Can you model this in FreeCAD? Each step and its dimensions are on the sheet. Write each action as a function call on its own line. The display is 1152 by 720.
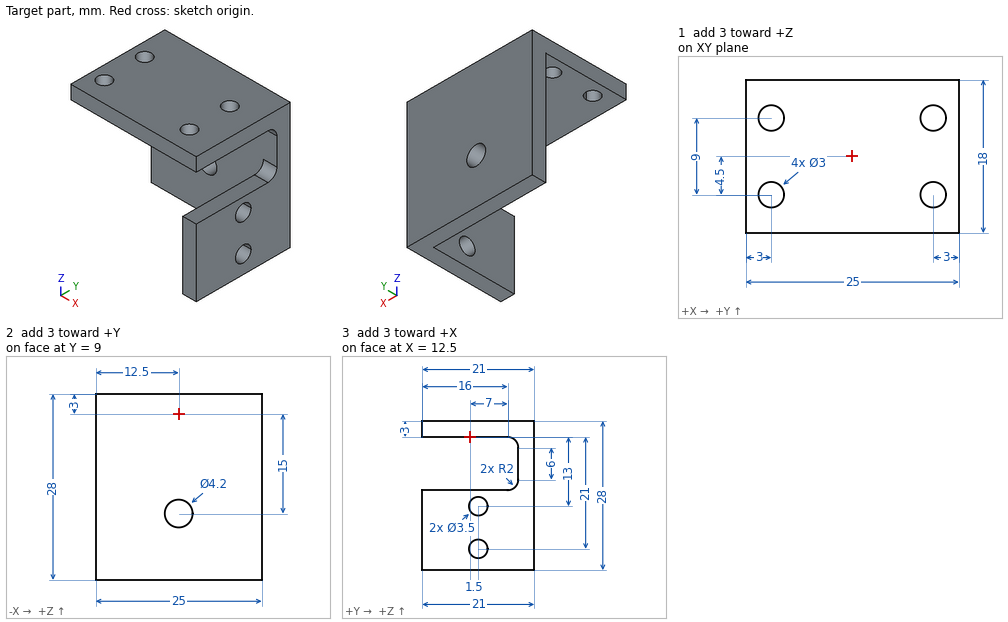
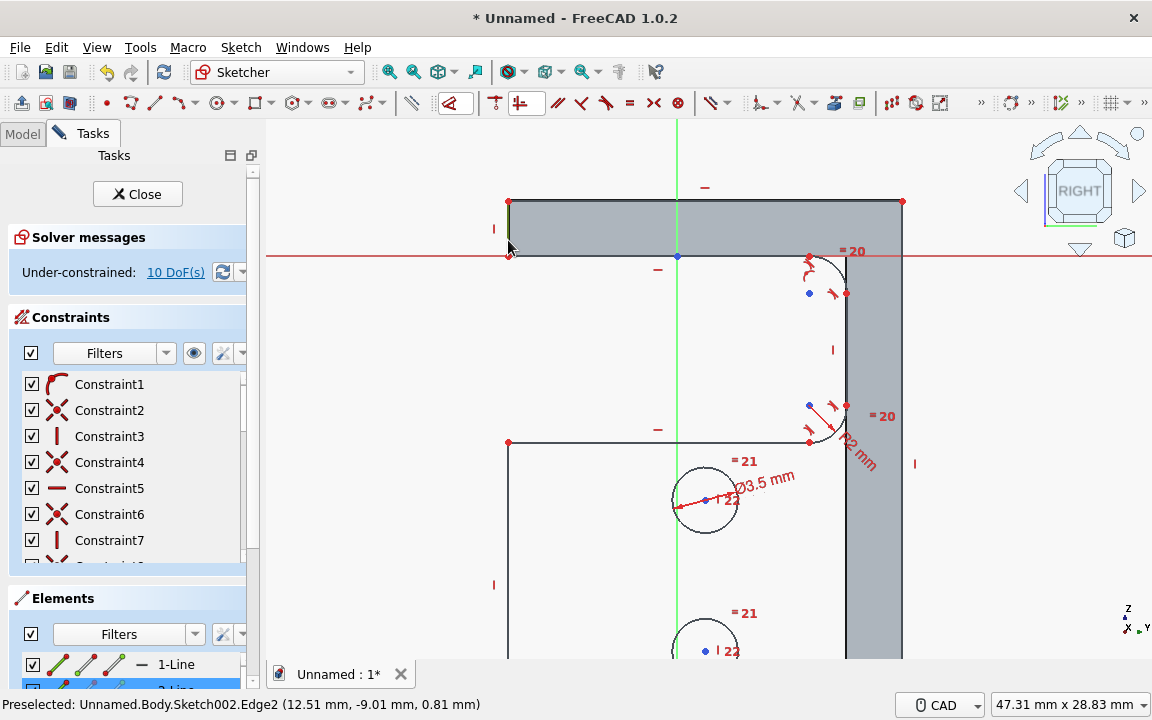
key(i)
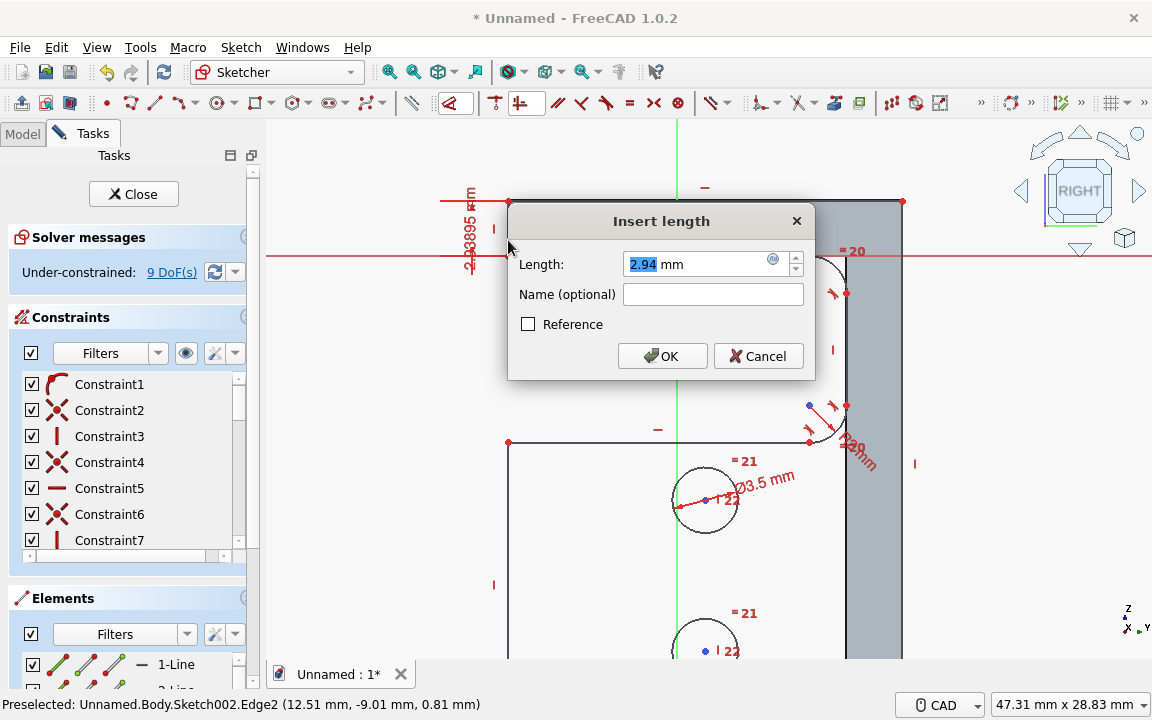
text(3)
key(Return)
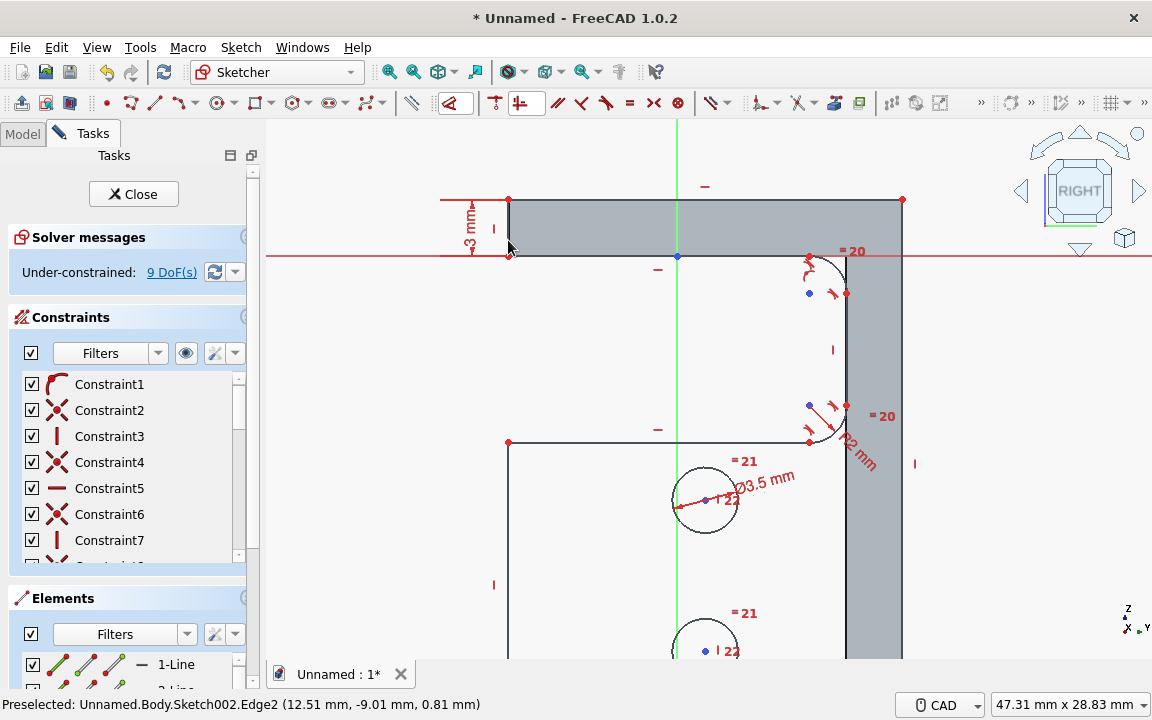
click(847, 372)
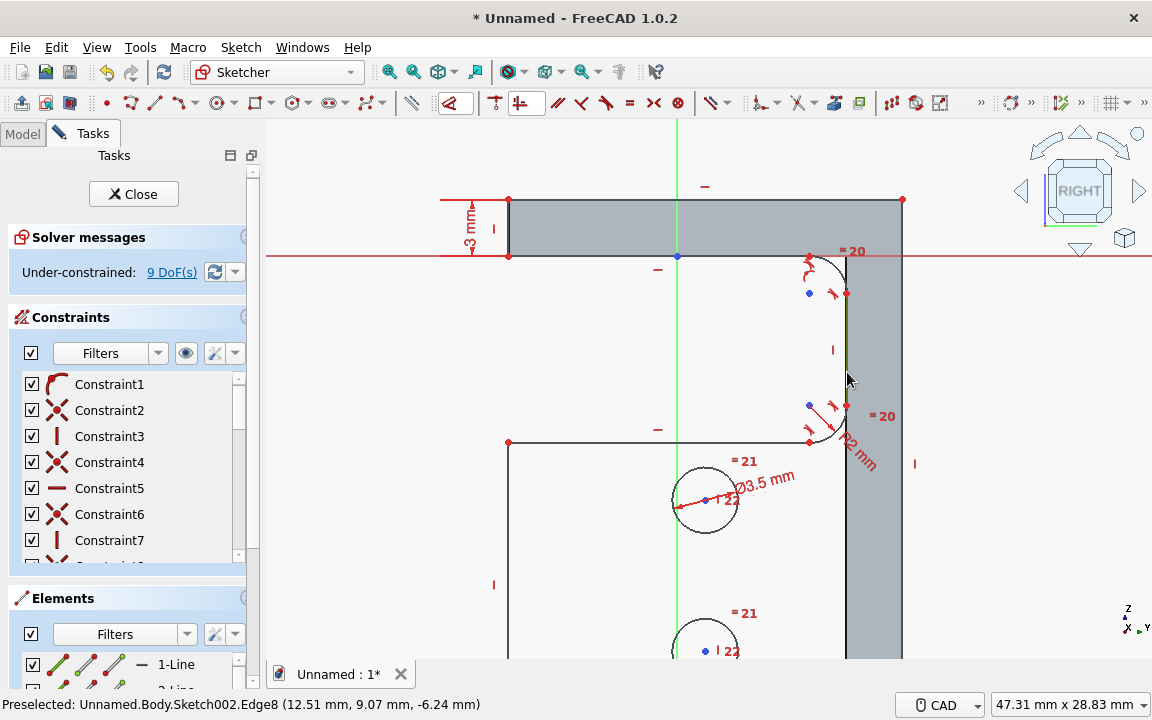
click(468, 104)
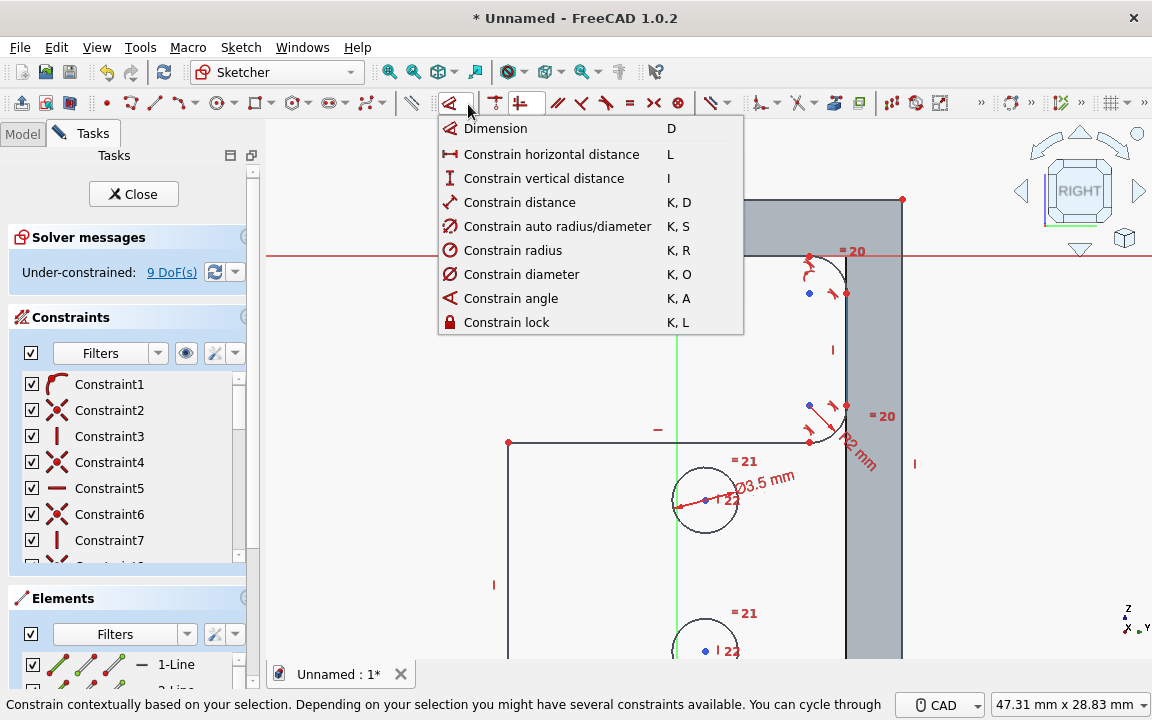
click(591, 178)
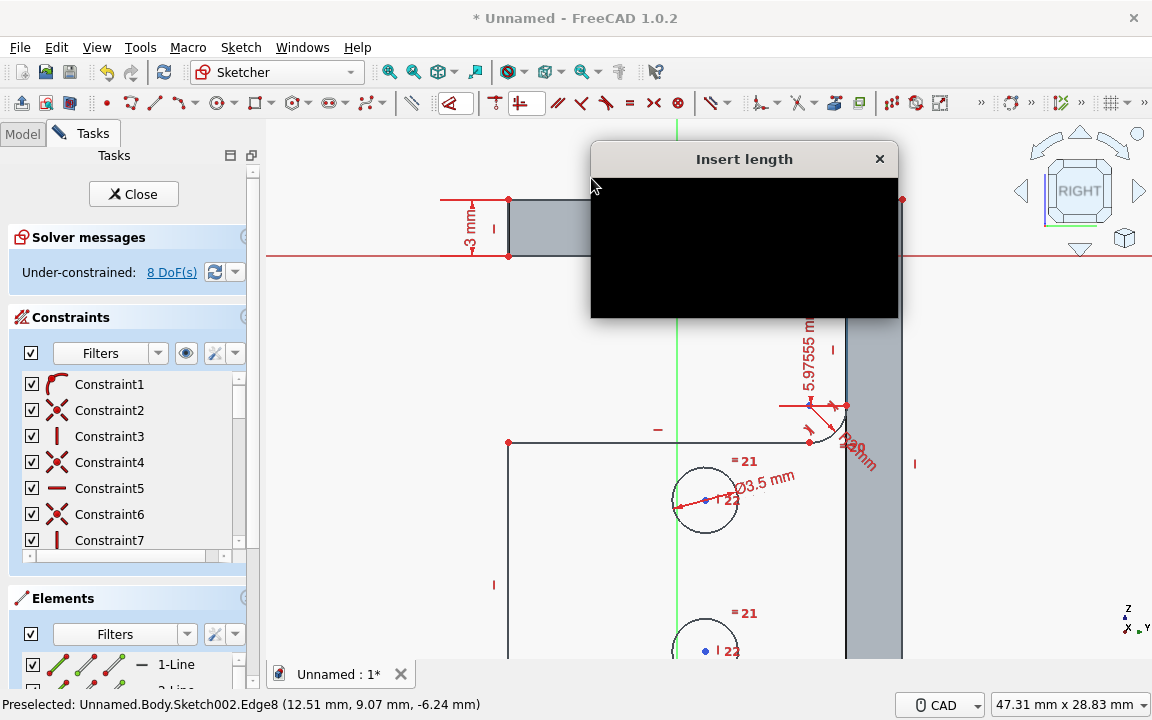
text(6)
key(Return)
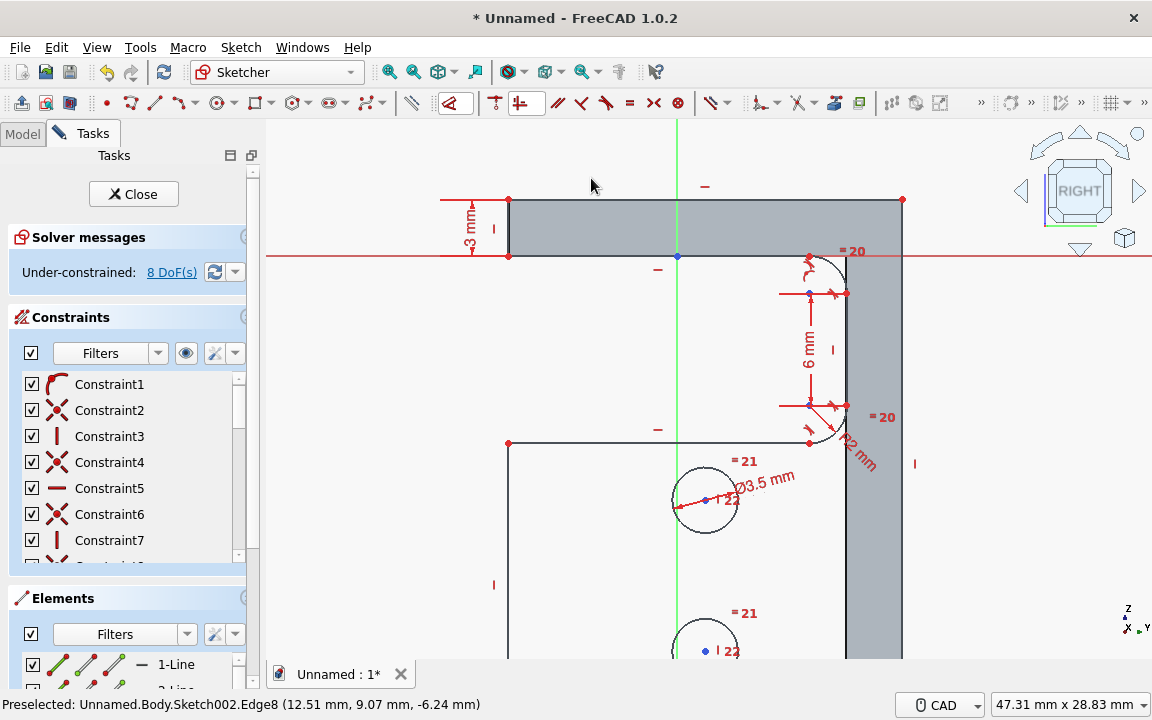
click(719, 256)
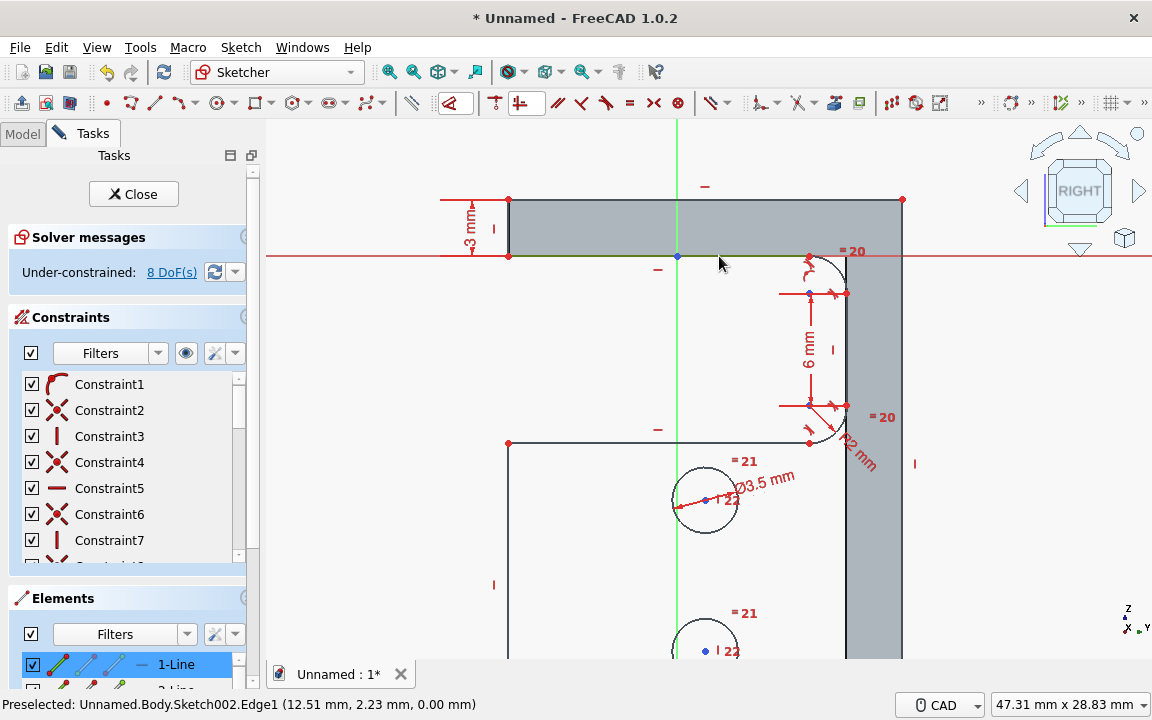
click(468, 104)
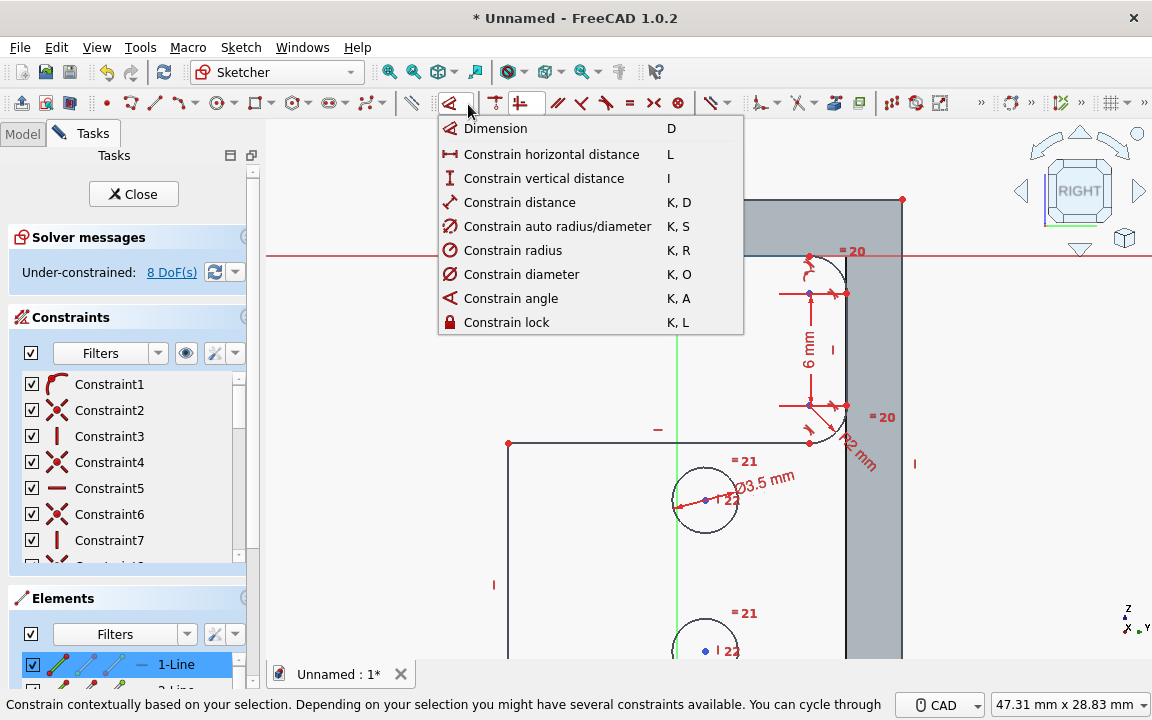
click(591, 154)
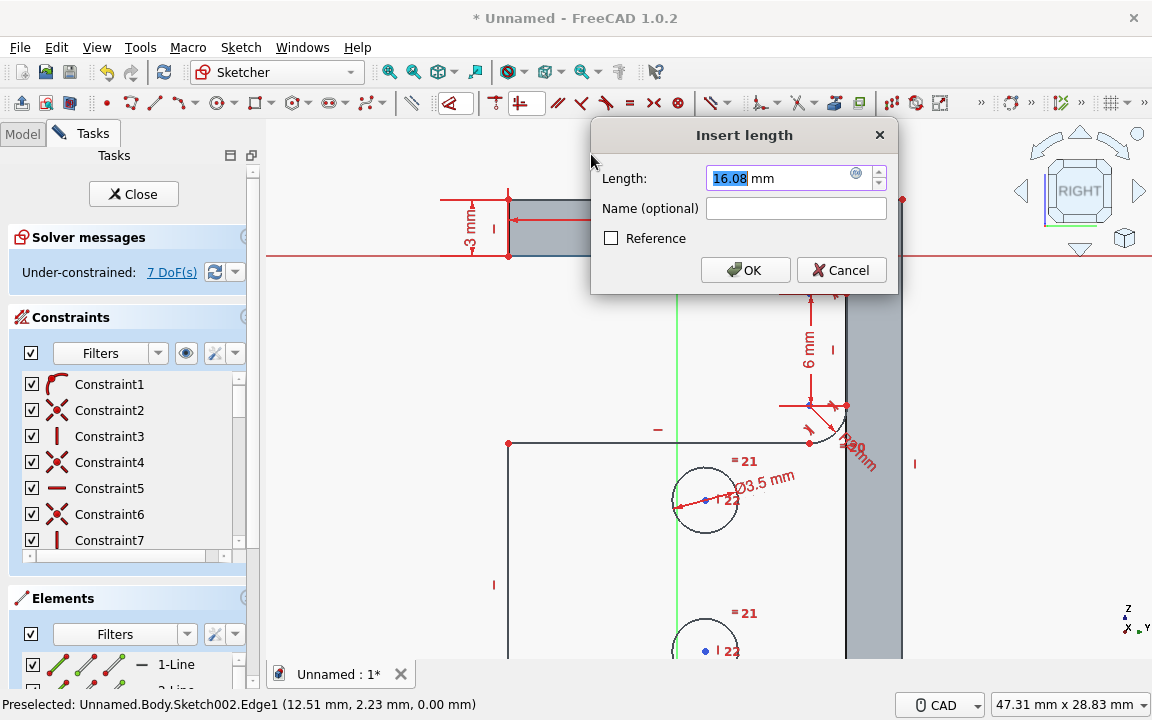
text(16)
key(Return)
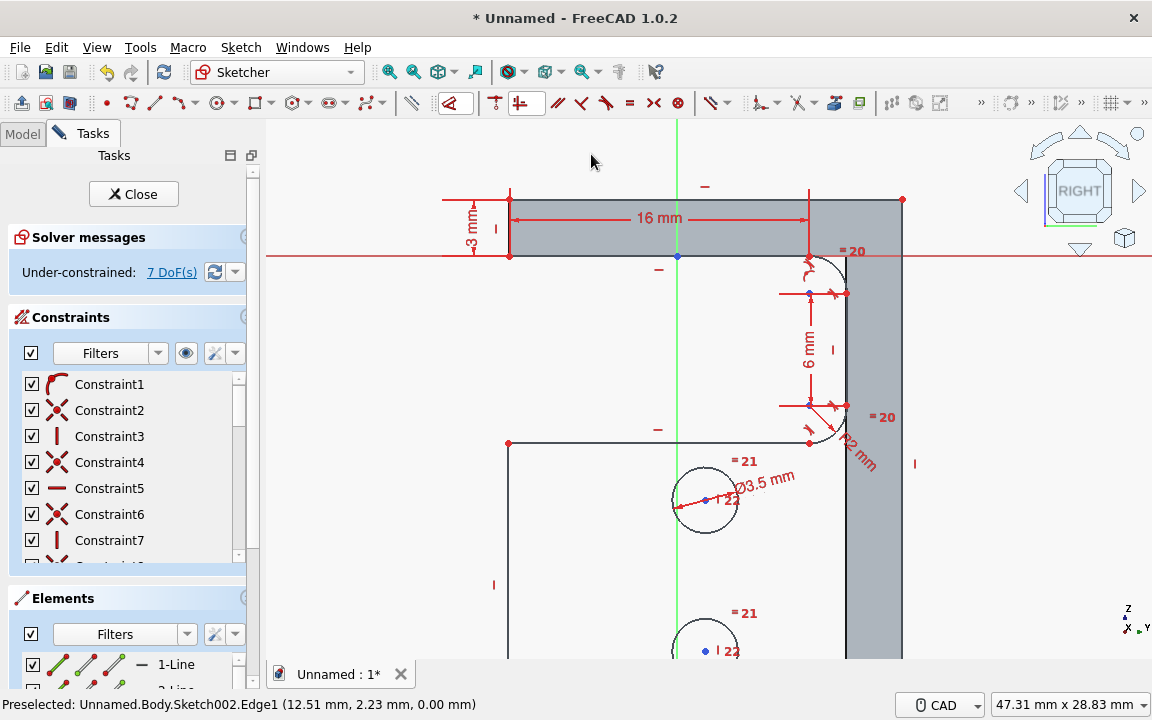
click(628, 200)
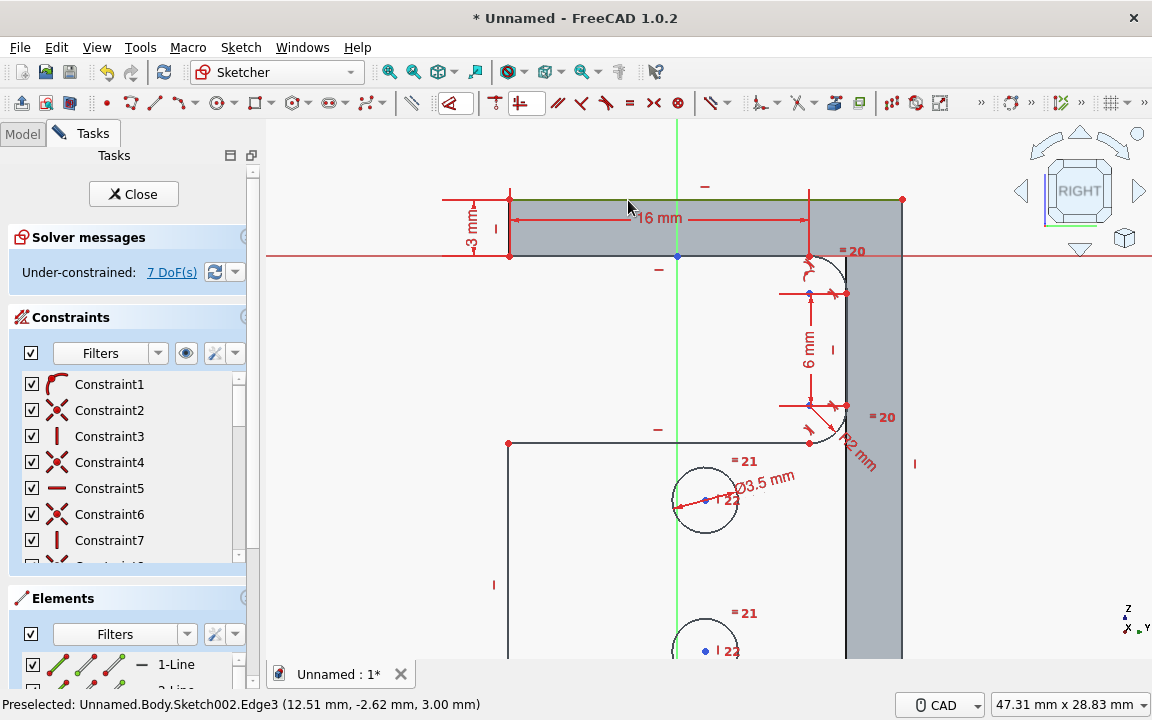
key(l)